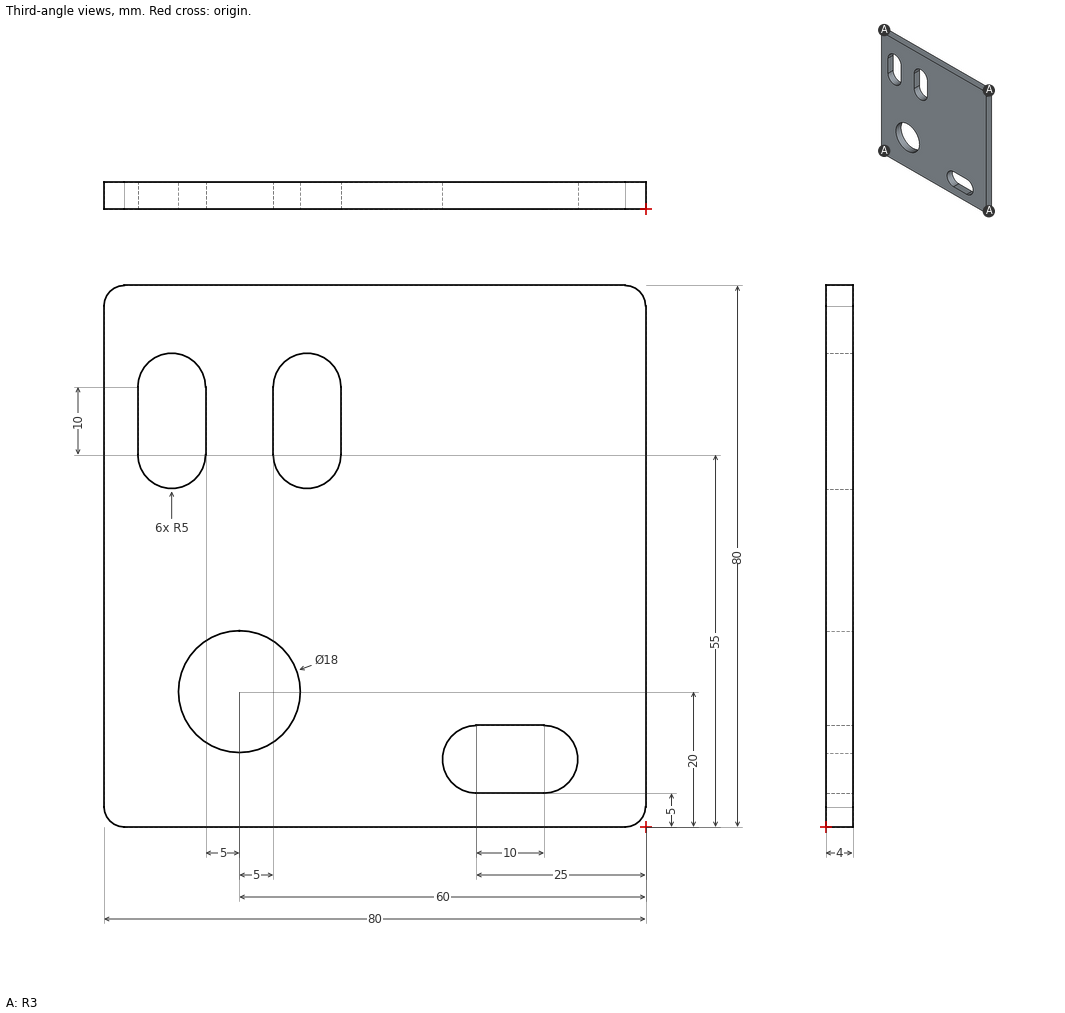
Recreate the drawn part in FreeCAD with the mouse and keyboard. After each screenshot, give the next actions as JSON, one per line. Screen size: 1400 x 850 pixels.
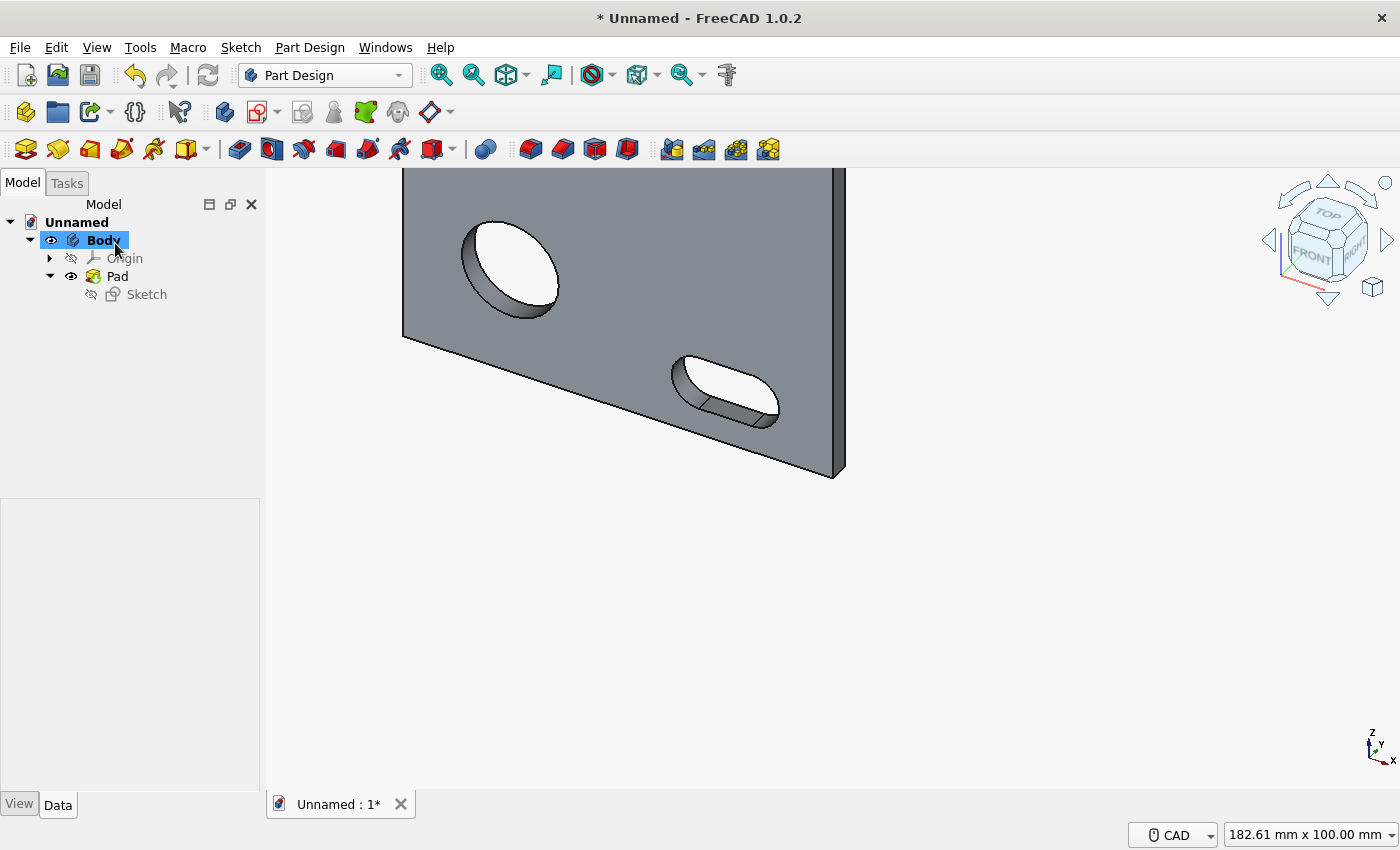
{"action": "left_click", "coordinate": [442, 76]}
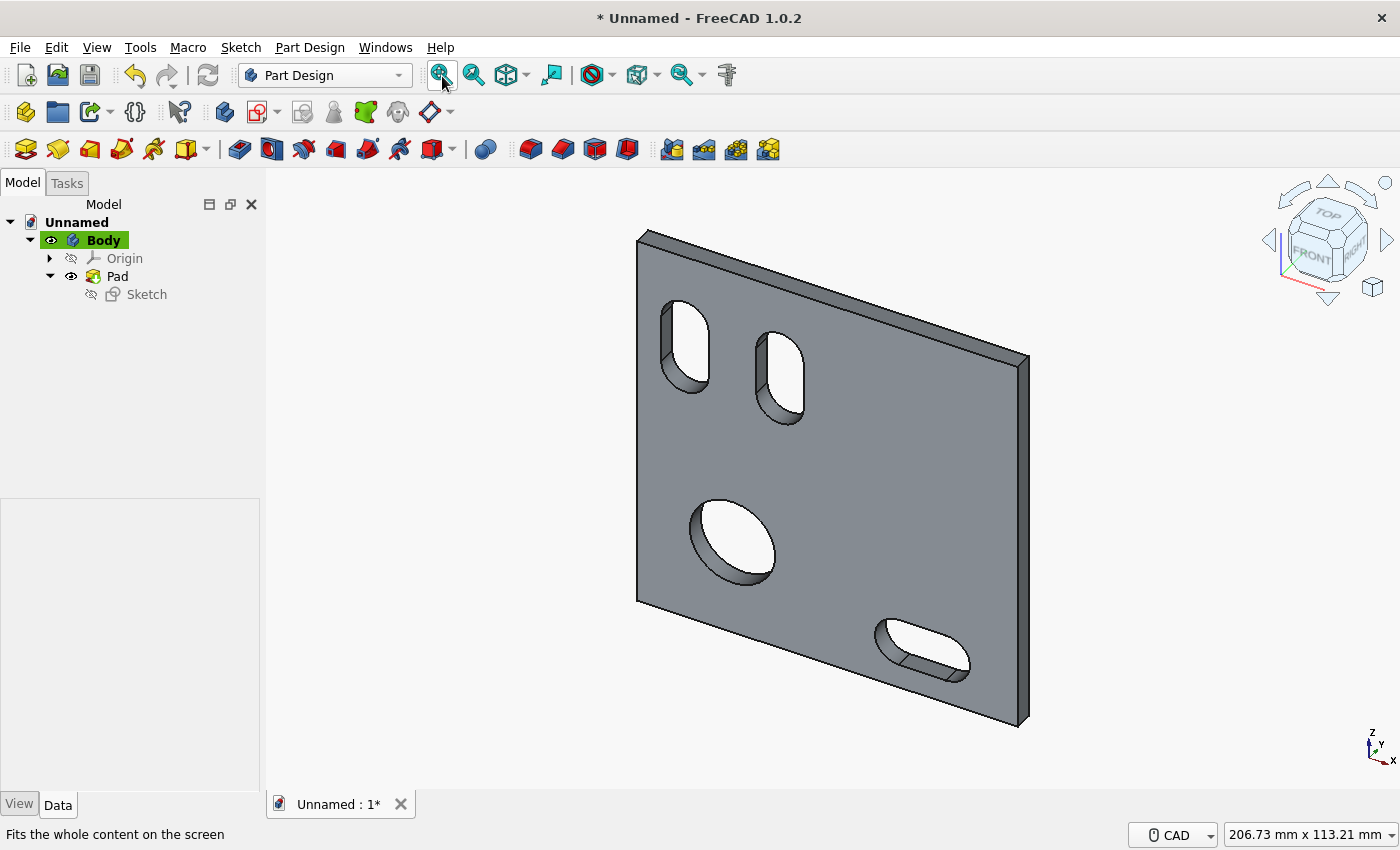
{"action": "left_click", "coordinate": [1023, 361]}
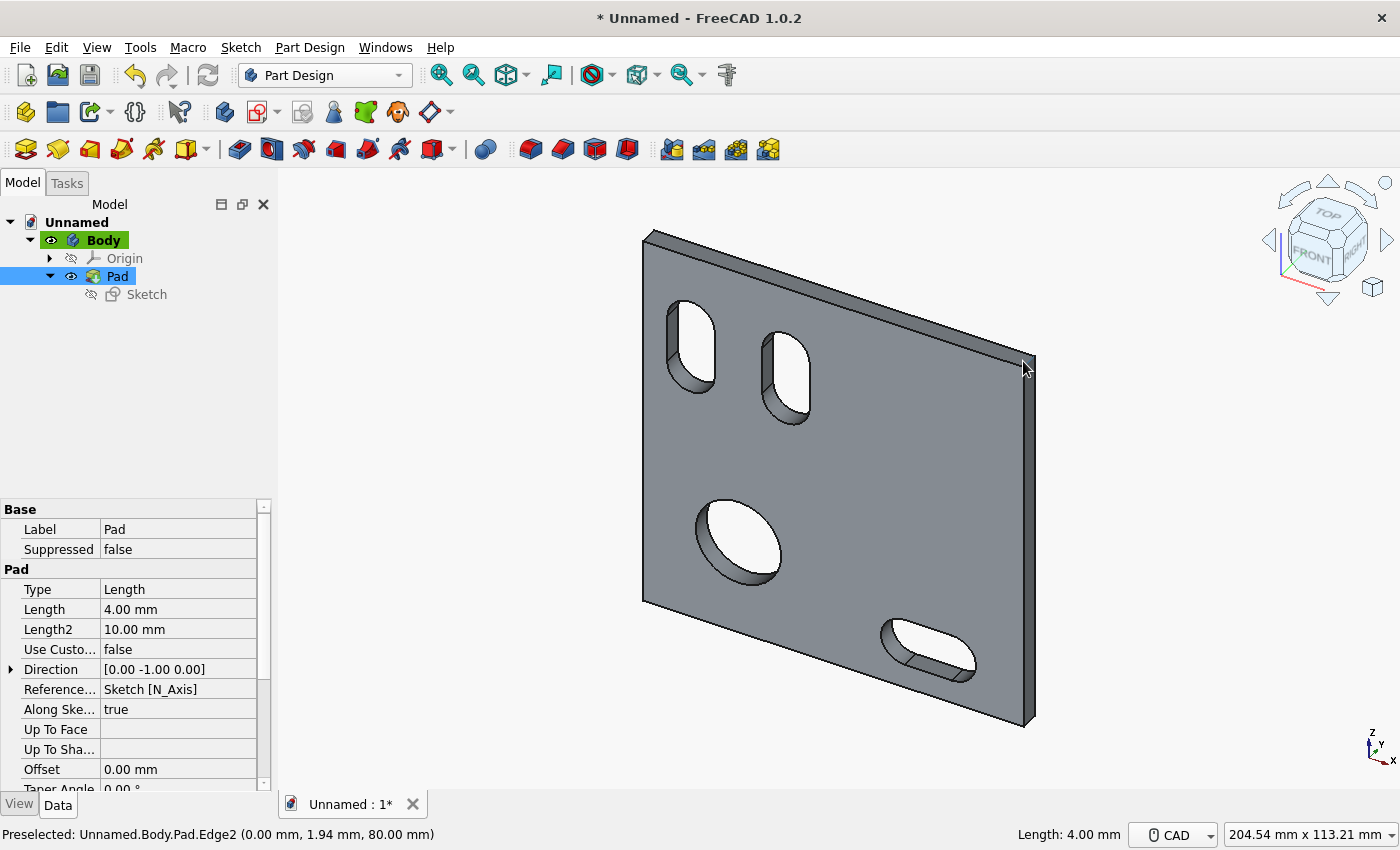
{"action": "scroll", "coordinate": [649, 235], "scroll_direction": "up", "scroll_amount": 4}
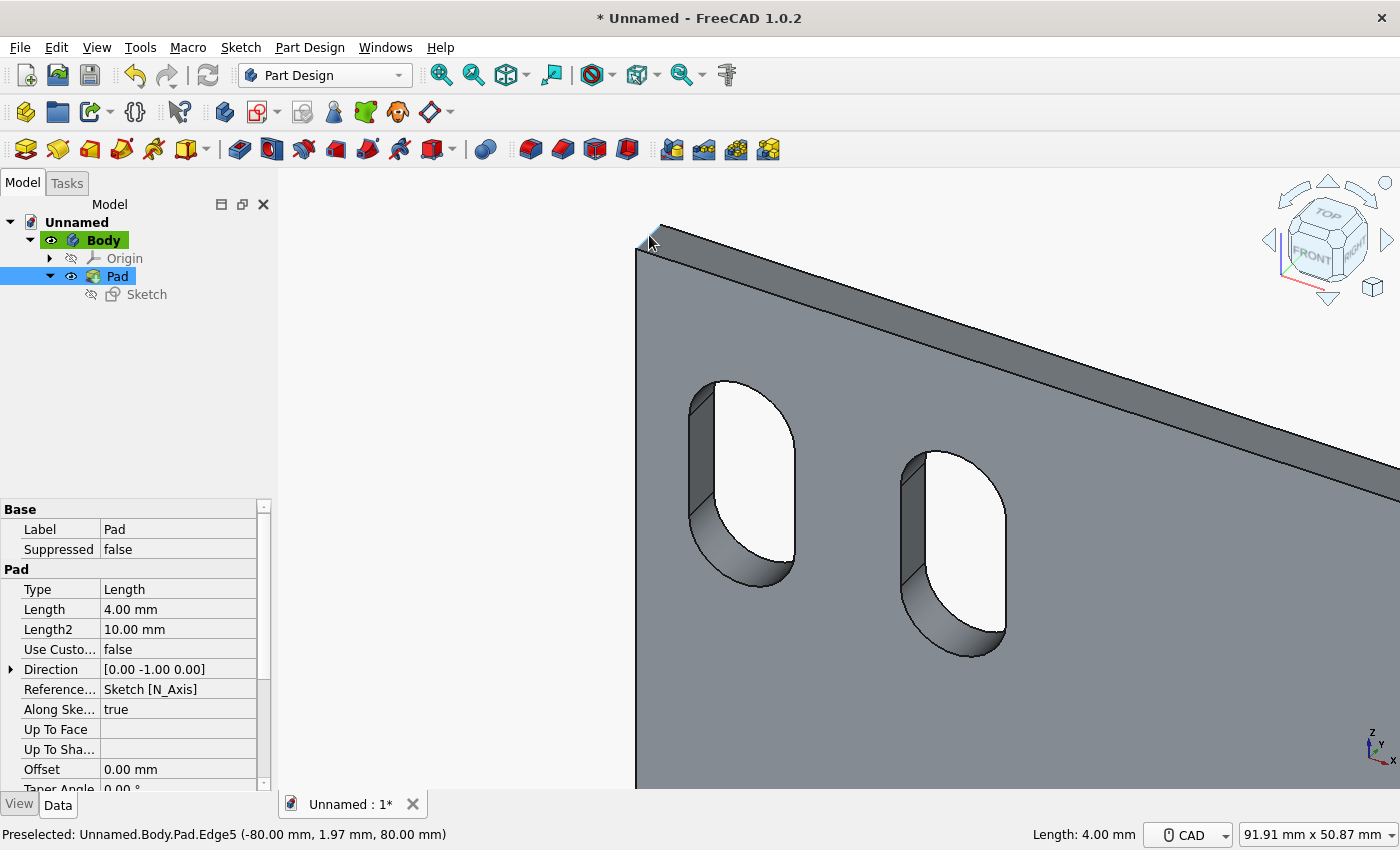
{"action": "left_click", "coordinate": [442, 76]}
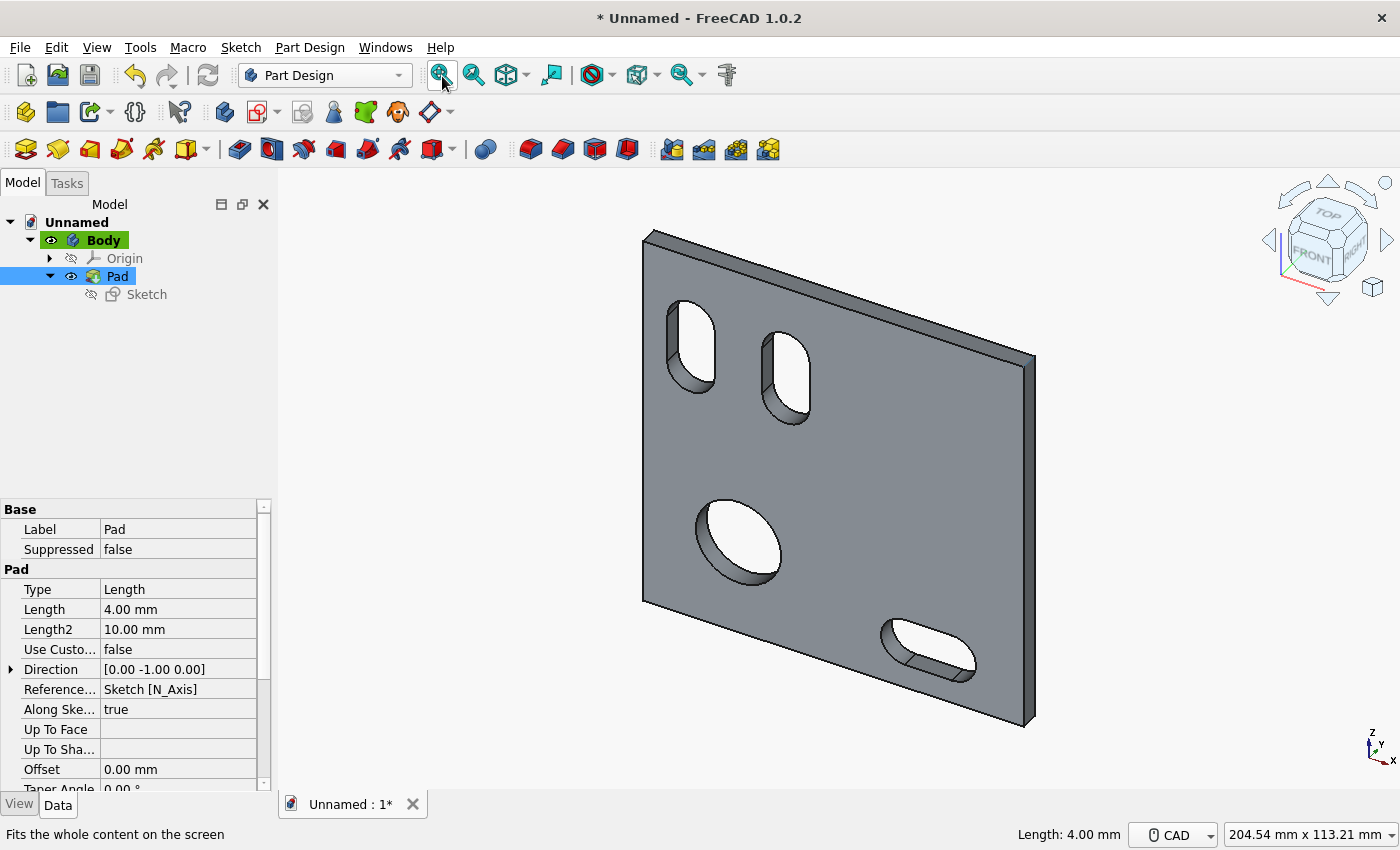
{"action": "key", "text": "0"}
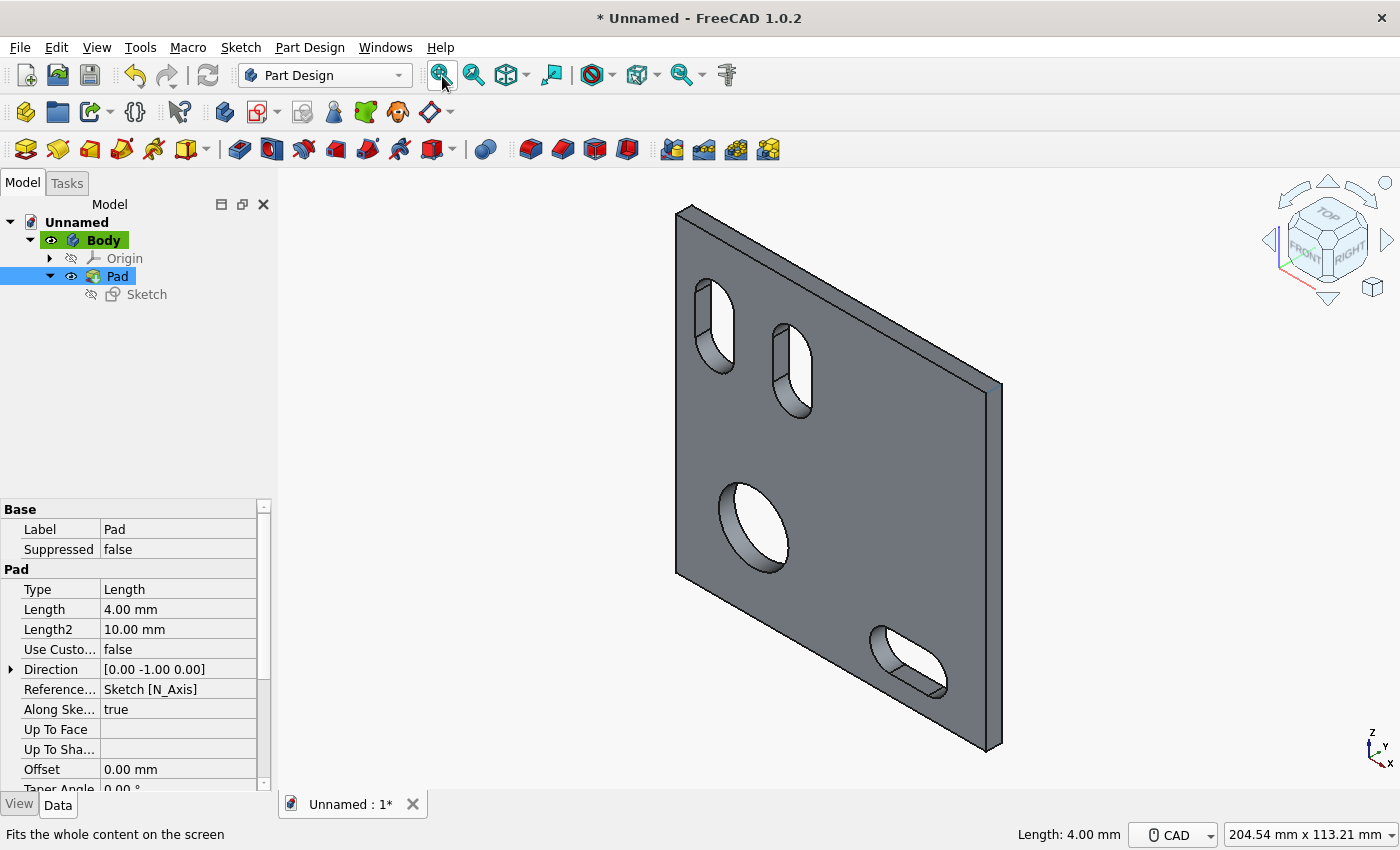
{"action": "scroll", "coordinate": [684, 209], "scroll_direction": "up", "scroll_amount": 4}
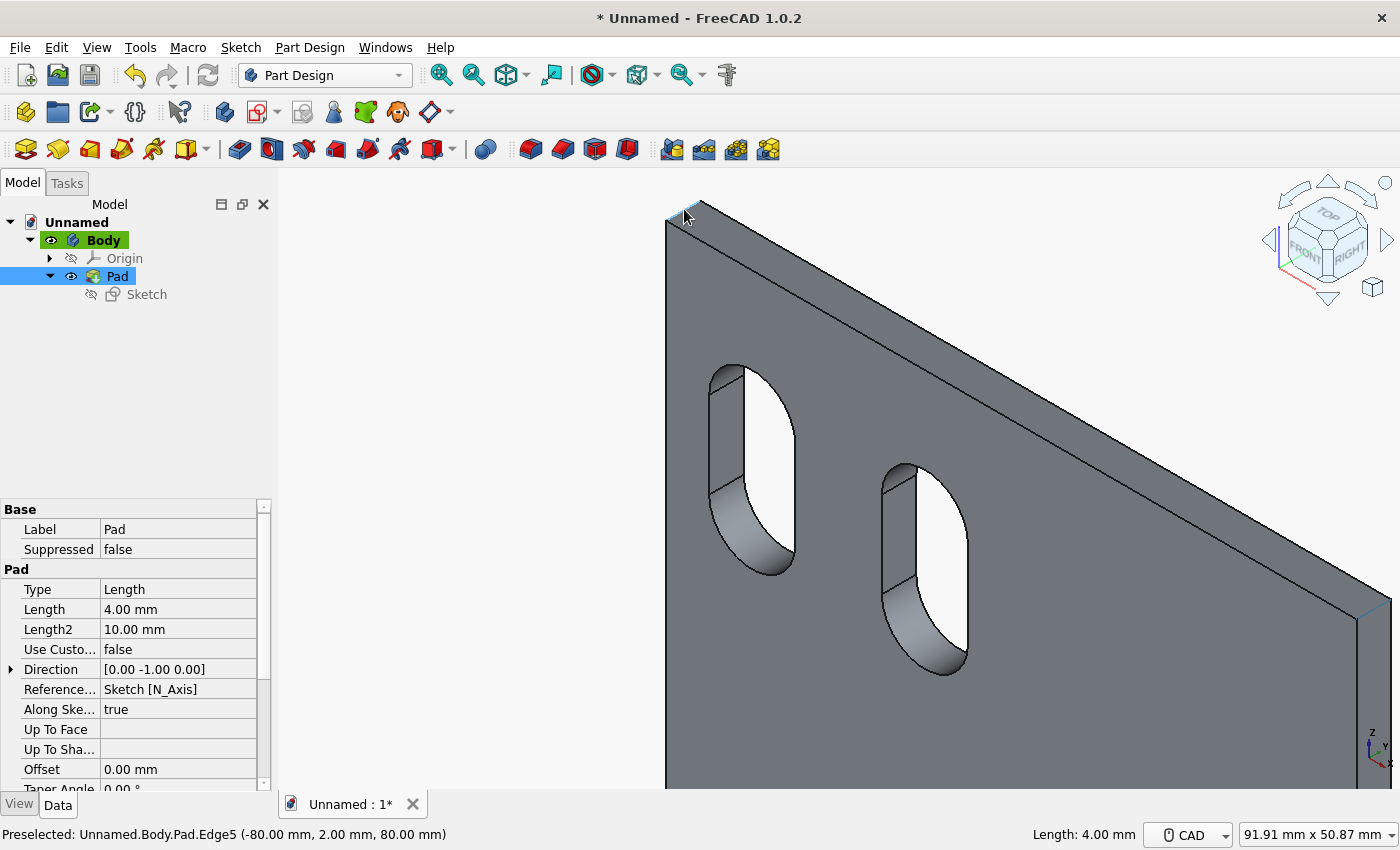
{"action": "left_click", "coordinate": [442, 76]}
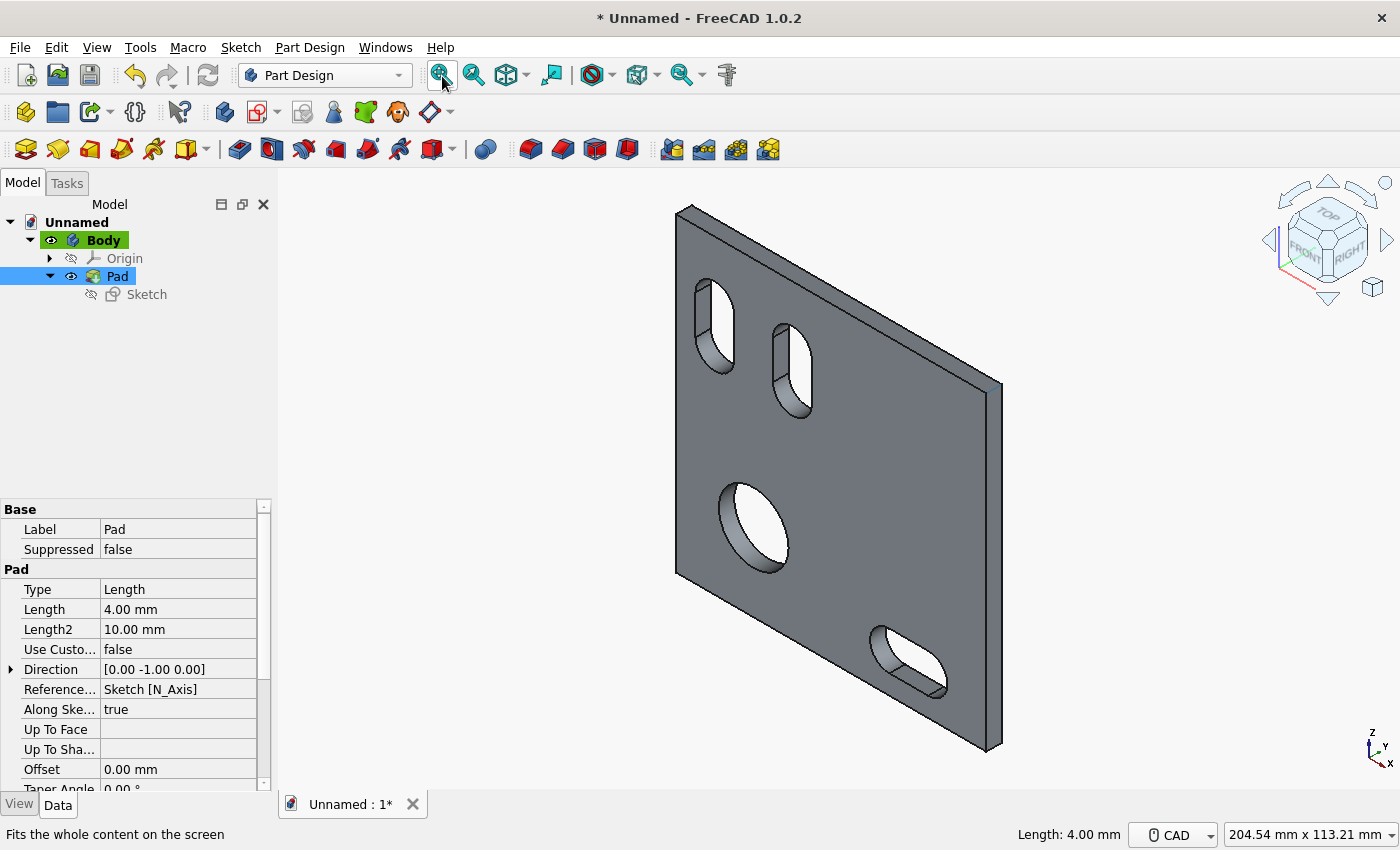
{"action": "key", "text": "2"}